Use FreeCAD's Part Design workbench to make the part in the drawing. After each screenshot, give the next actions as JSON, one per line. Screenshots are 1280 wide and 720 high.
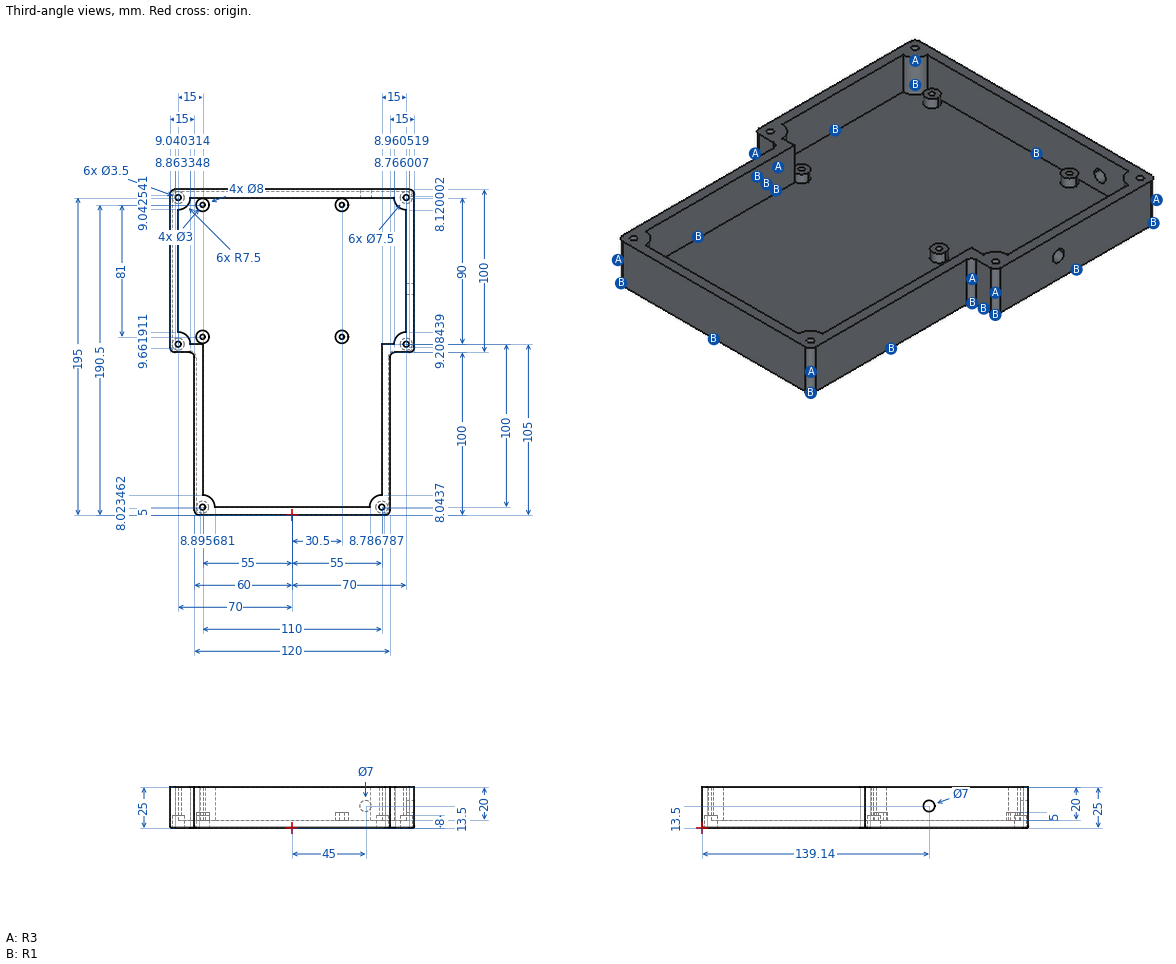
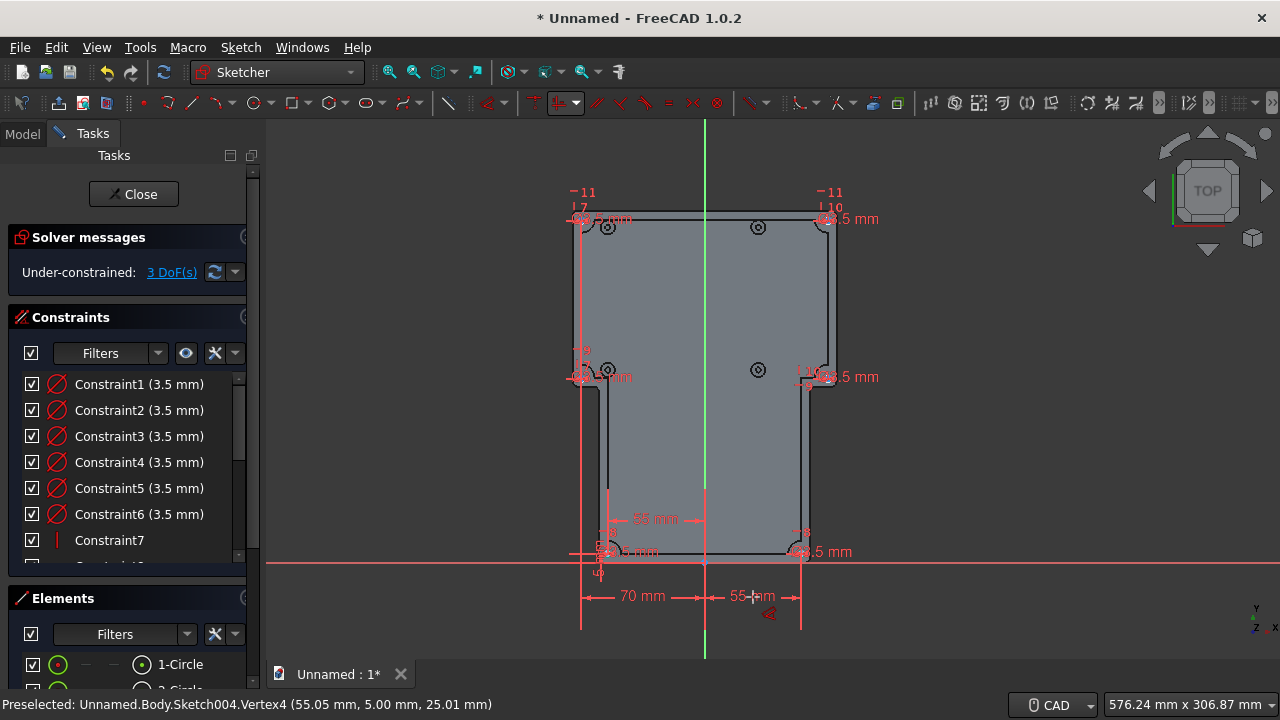
{"action": "left_click", "coordinate": [828, 379]}
{"action": "left_click", "coordinate": [766, 345]}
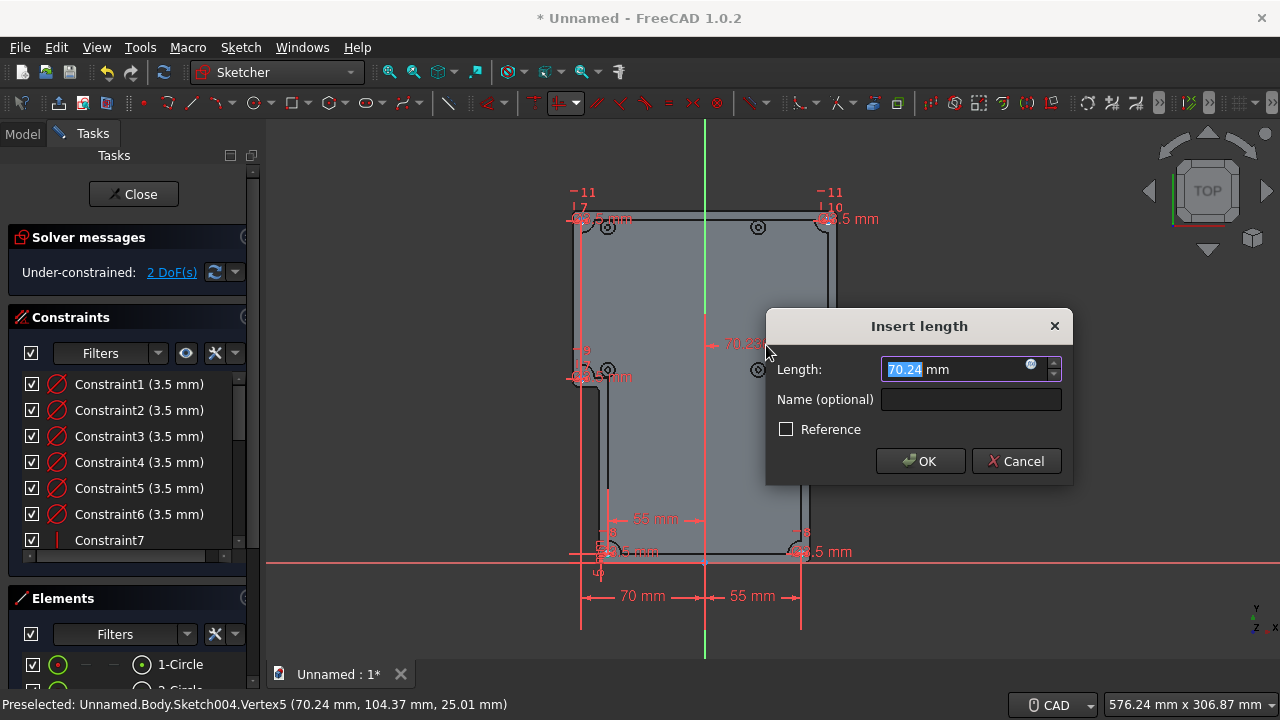
{"action": "type", "text": "70"}
{"action": "key", "text": "Return"}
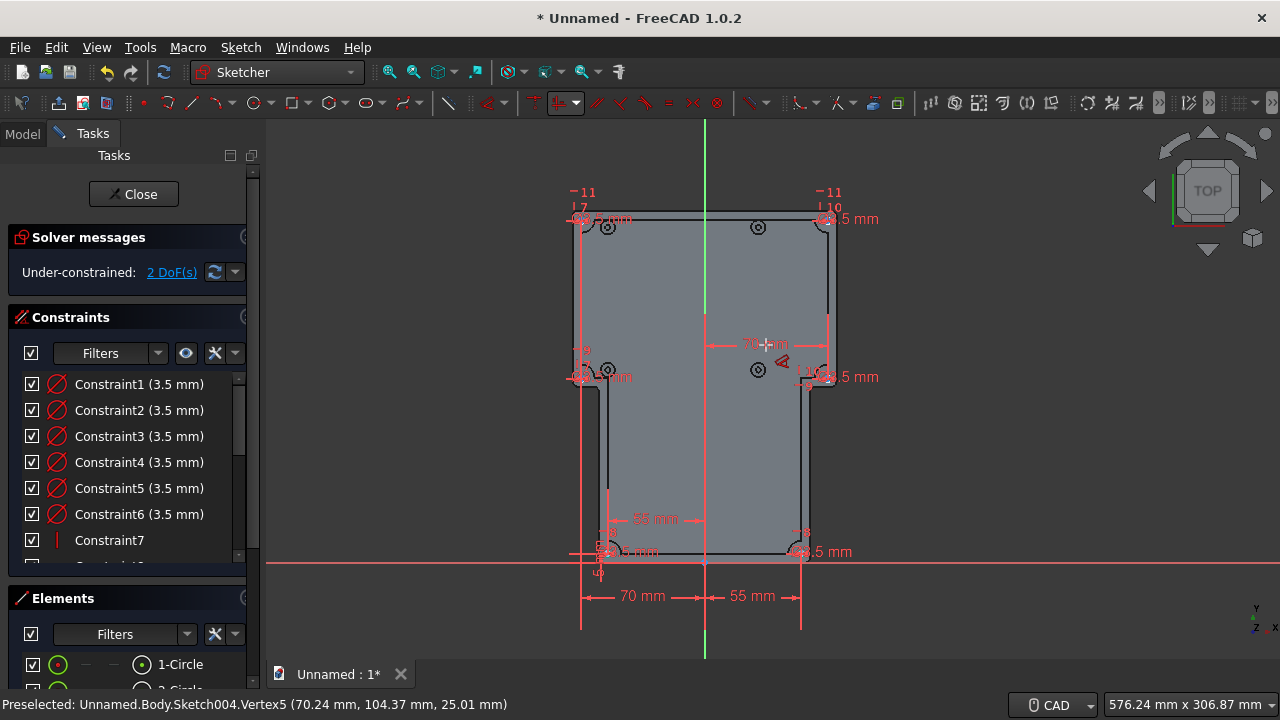
{"action": "left_click", "coordinate": [581, 221]}
{"action": "left_click", "coordinate": [547, 392]}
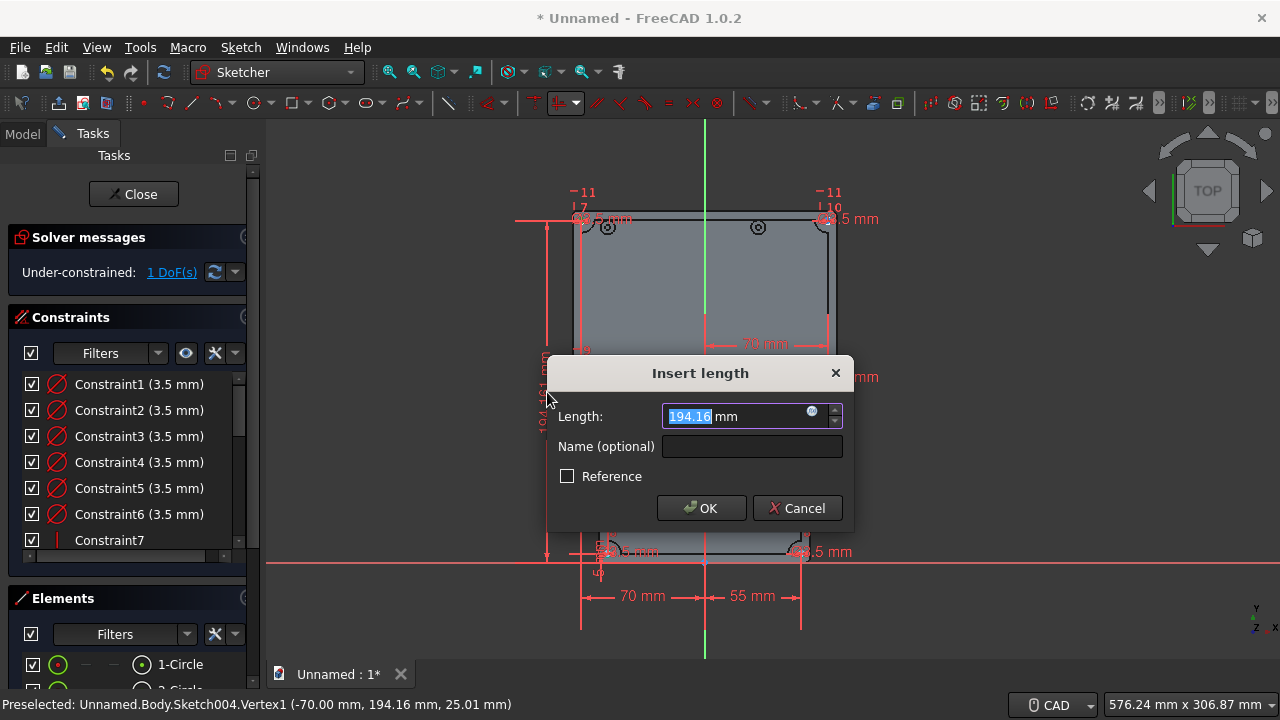
{"action": "type", "text": "195"}
{"action": "key", "text": "Return"}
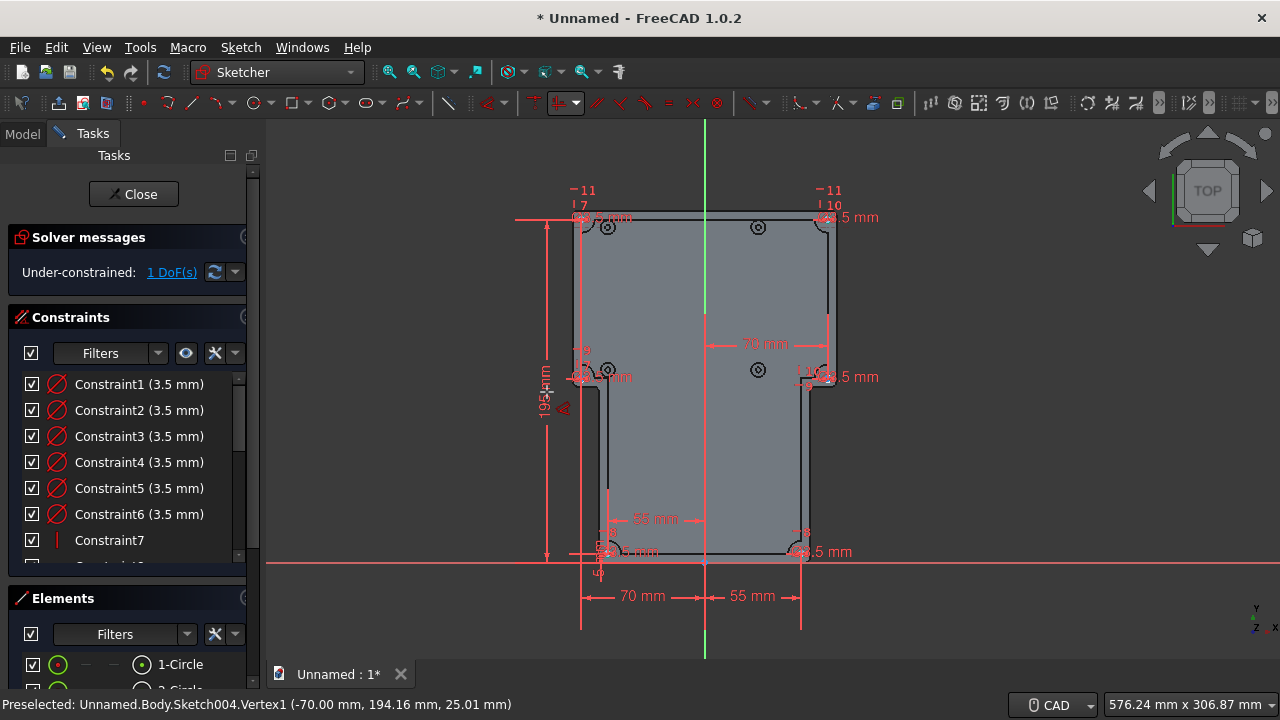
{"action": "left_click", "coordinate": [581, 379]}
{"action": "left_click", "coordinate": [547, 471]}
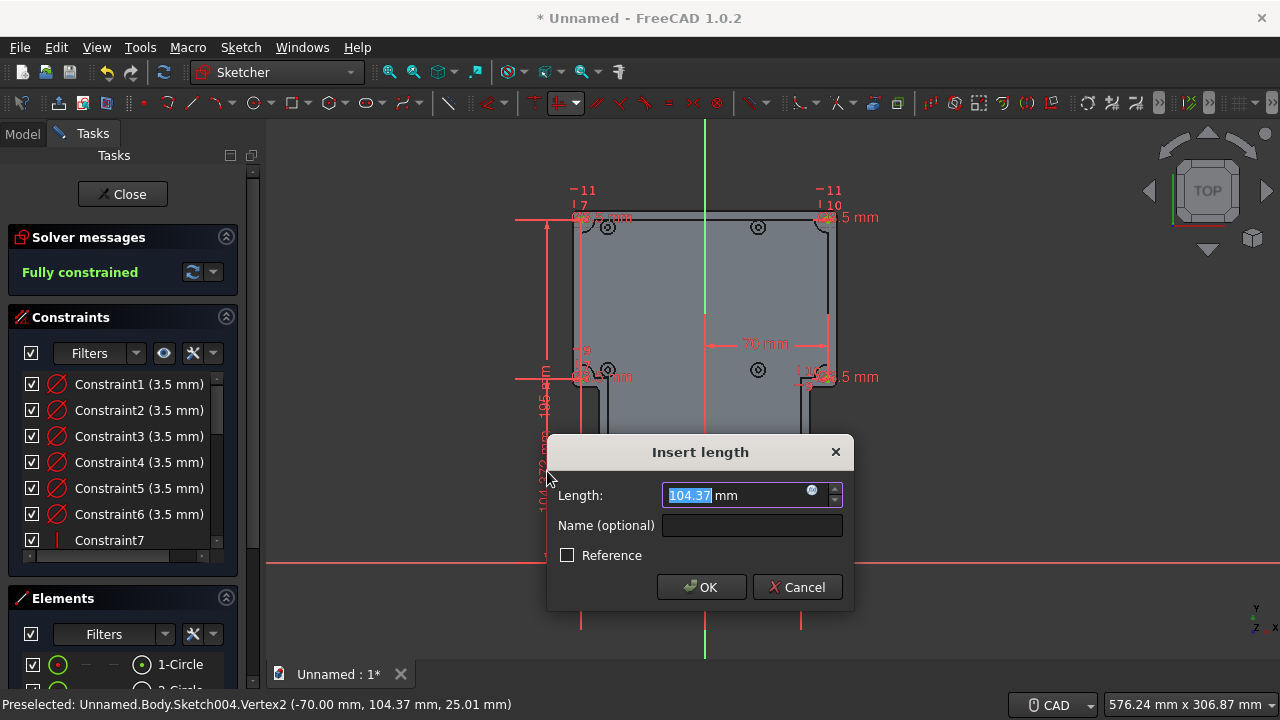
{"action": "type", "text": "105"}
{"action": "key", "text": "Return"}
{"action": "key", "text": "Escape"}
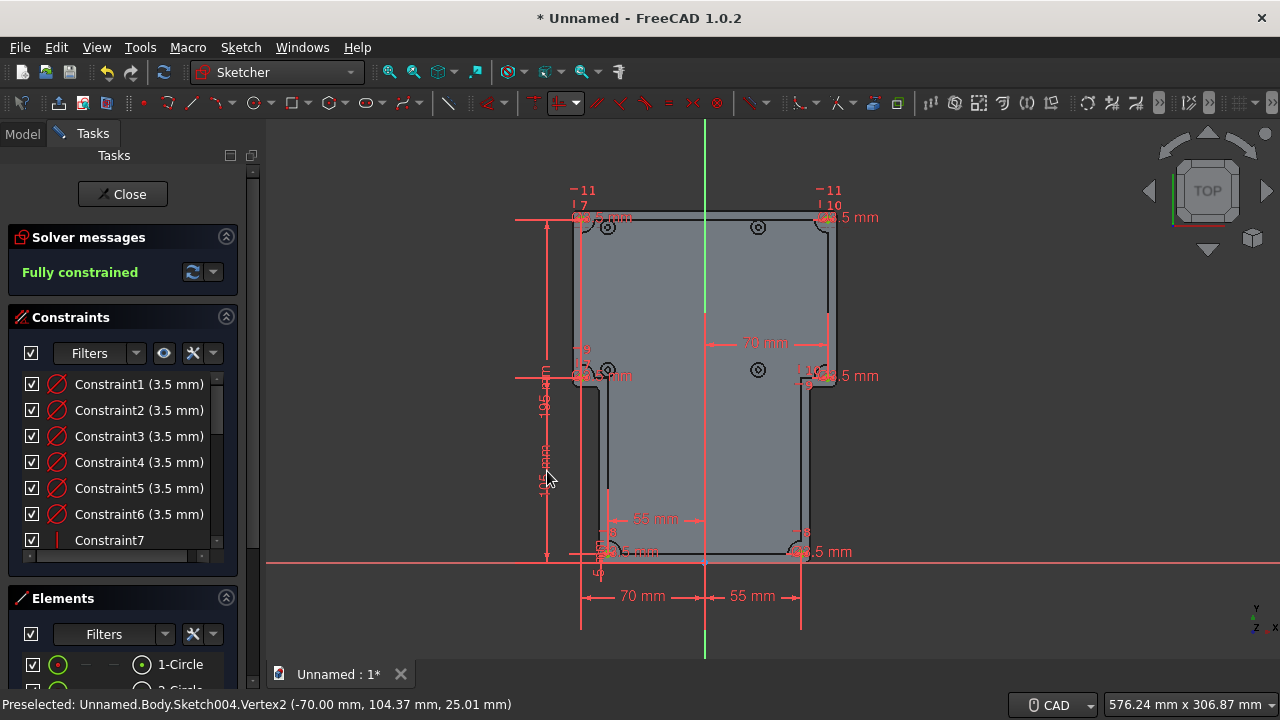
{"action": "left_click", "coordinate": [123, 194]}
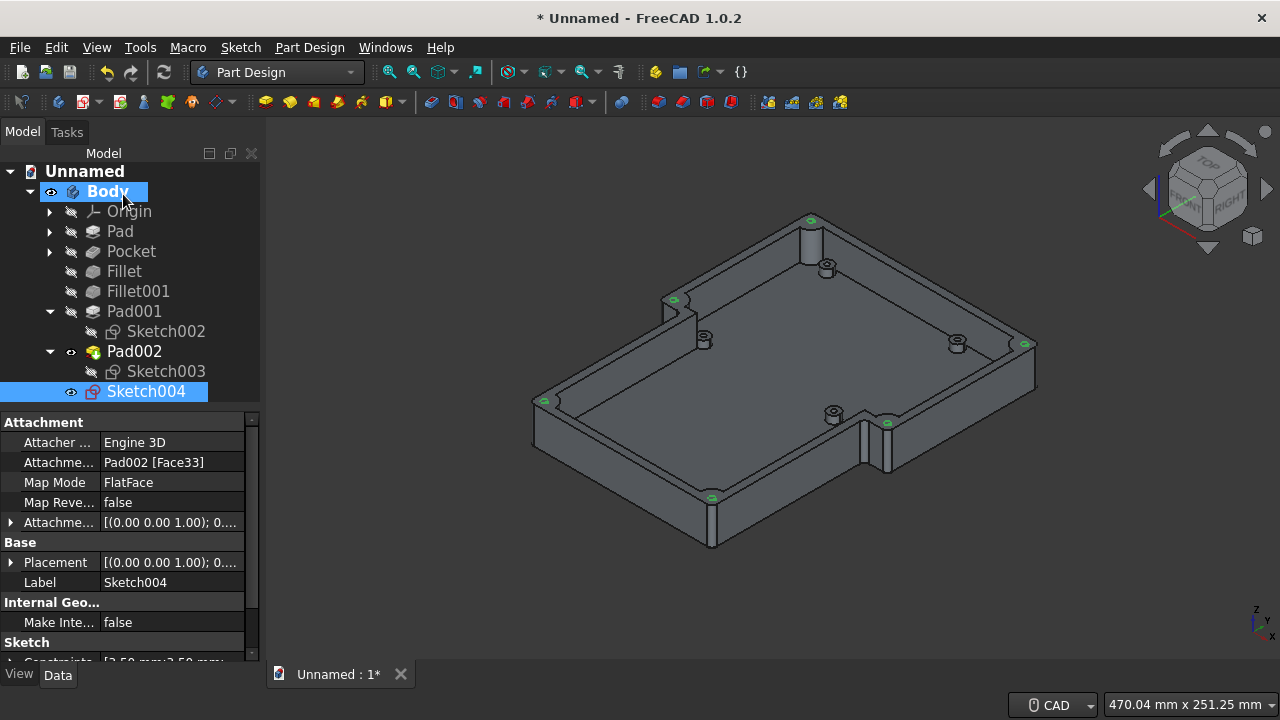
{"action": "left_click", "coordinate": [432, 102]}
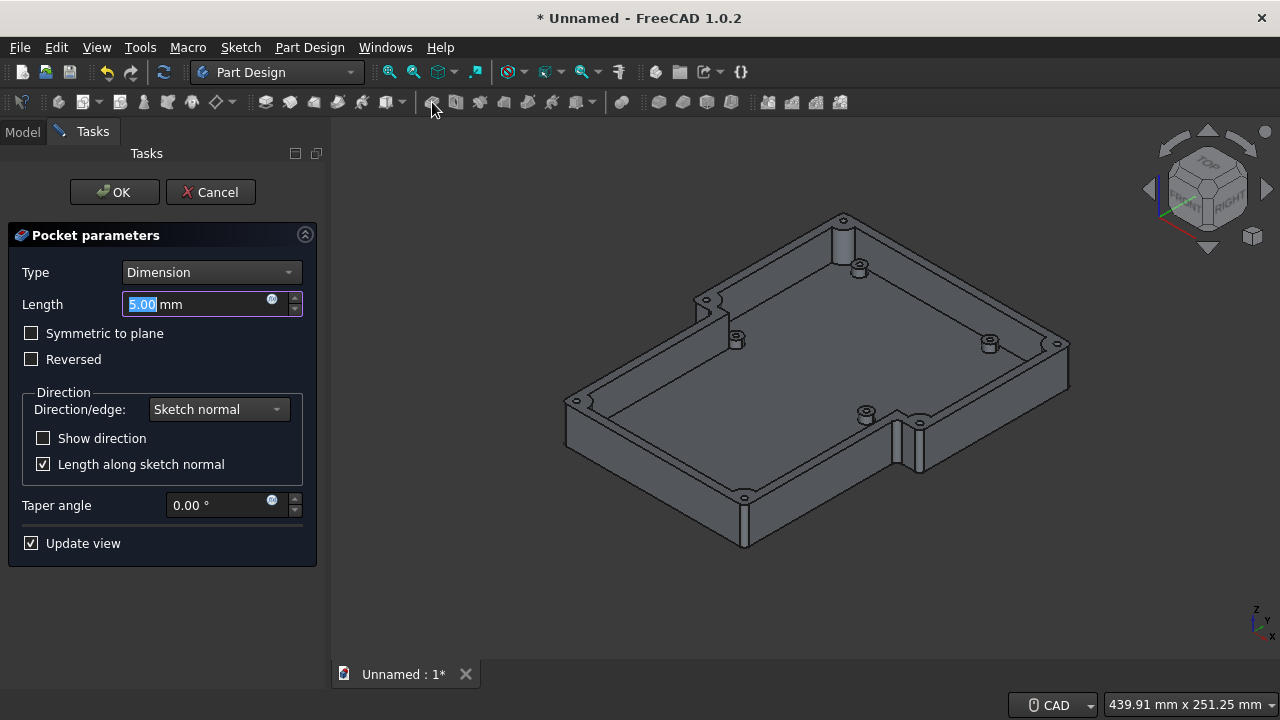
{"action": "type", "text": "20"}
{"action": "key", "text": "Tab"}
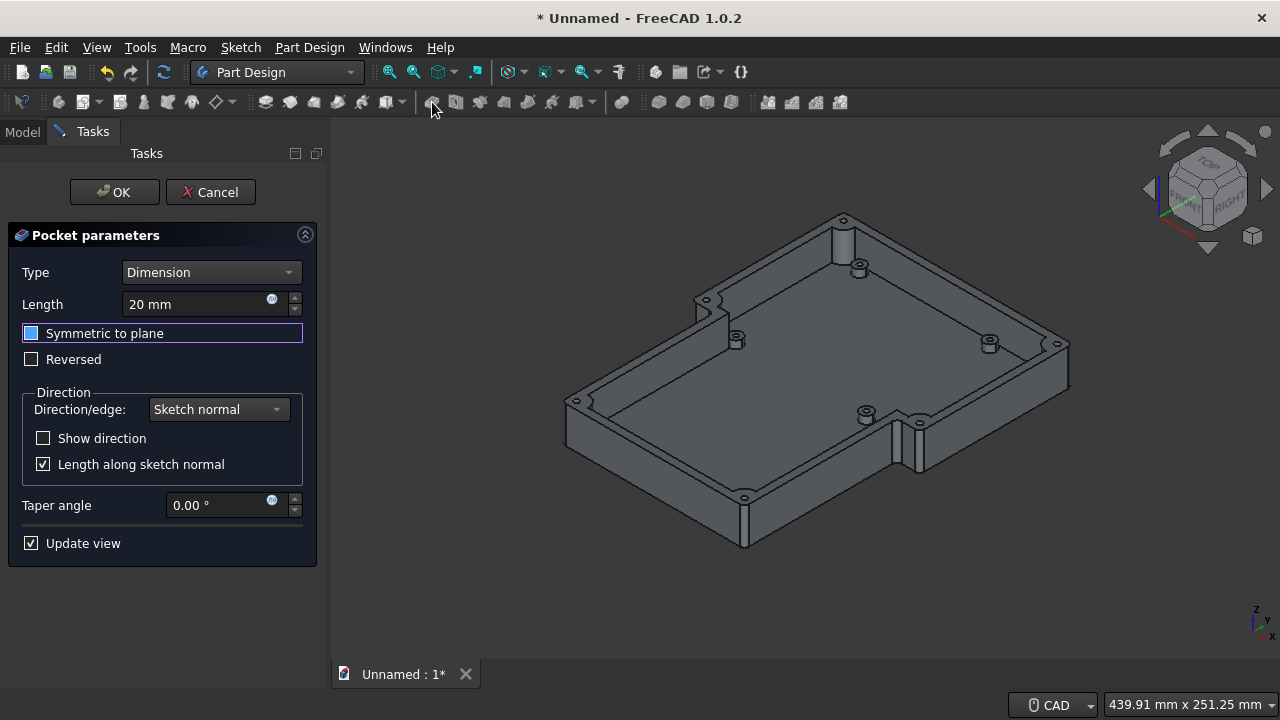
{"action": "left_click", "coordinate": [115, 192]}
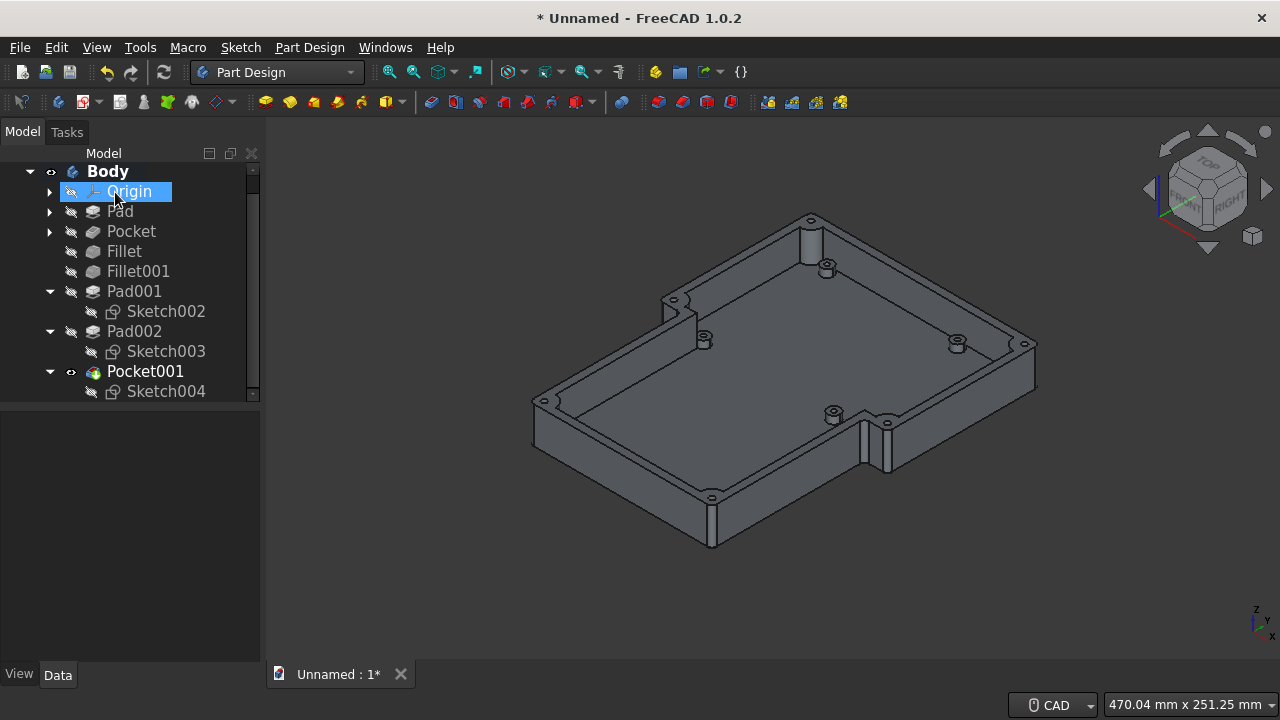
{"action": "key", "text": "5"}